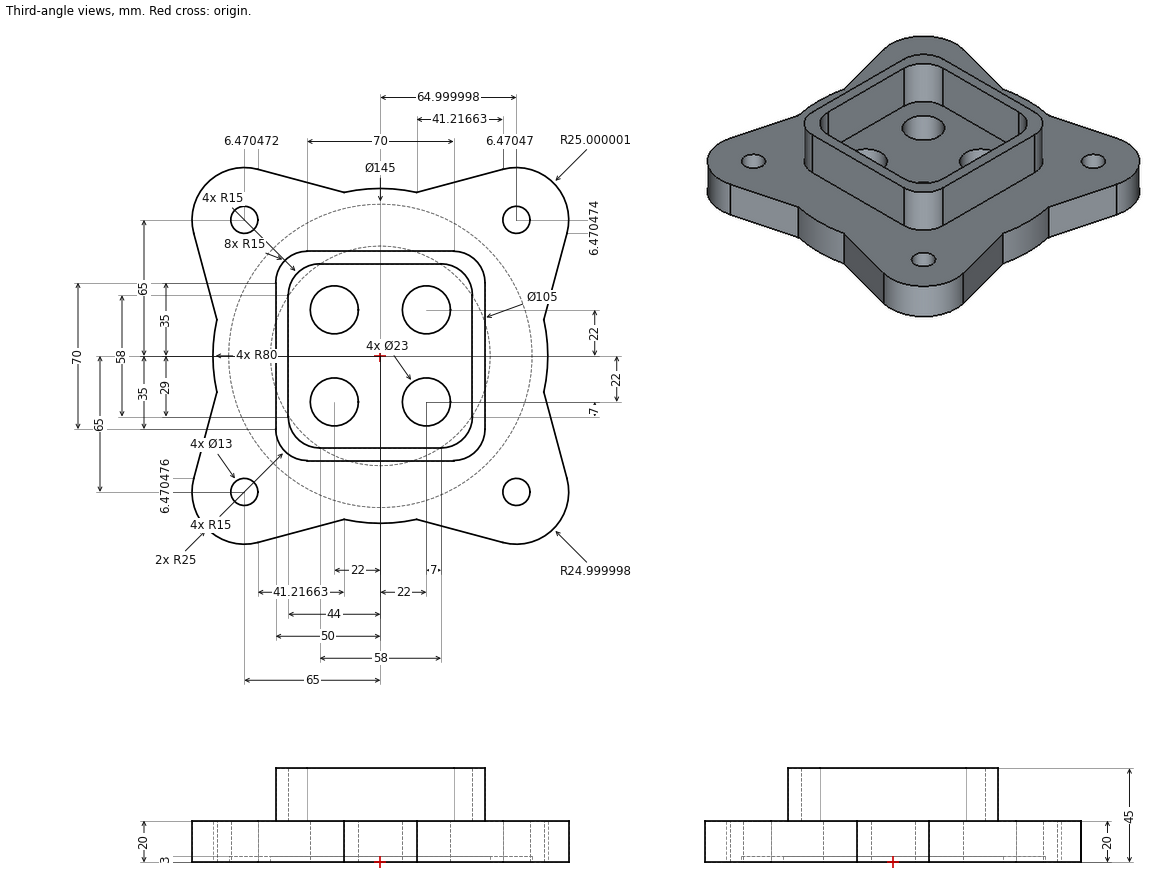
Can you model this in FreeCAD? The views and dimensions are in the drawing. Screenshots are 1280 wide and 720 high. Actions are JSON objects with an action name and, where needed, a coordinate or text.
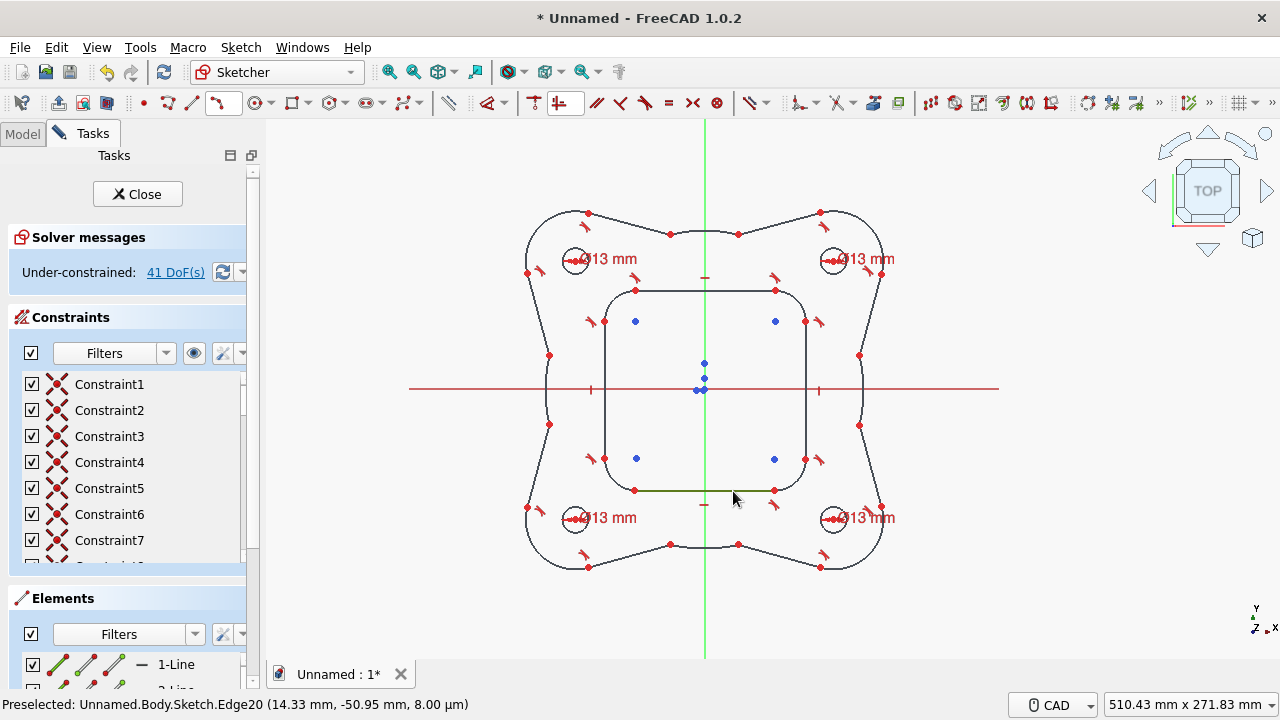
{"action": "left_click", "coordinate": [608, 473]}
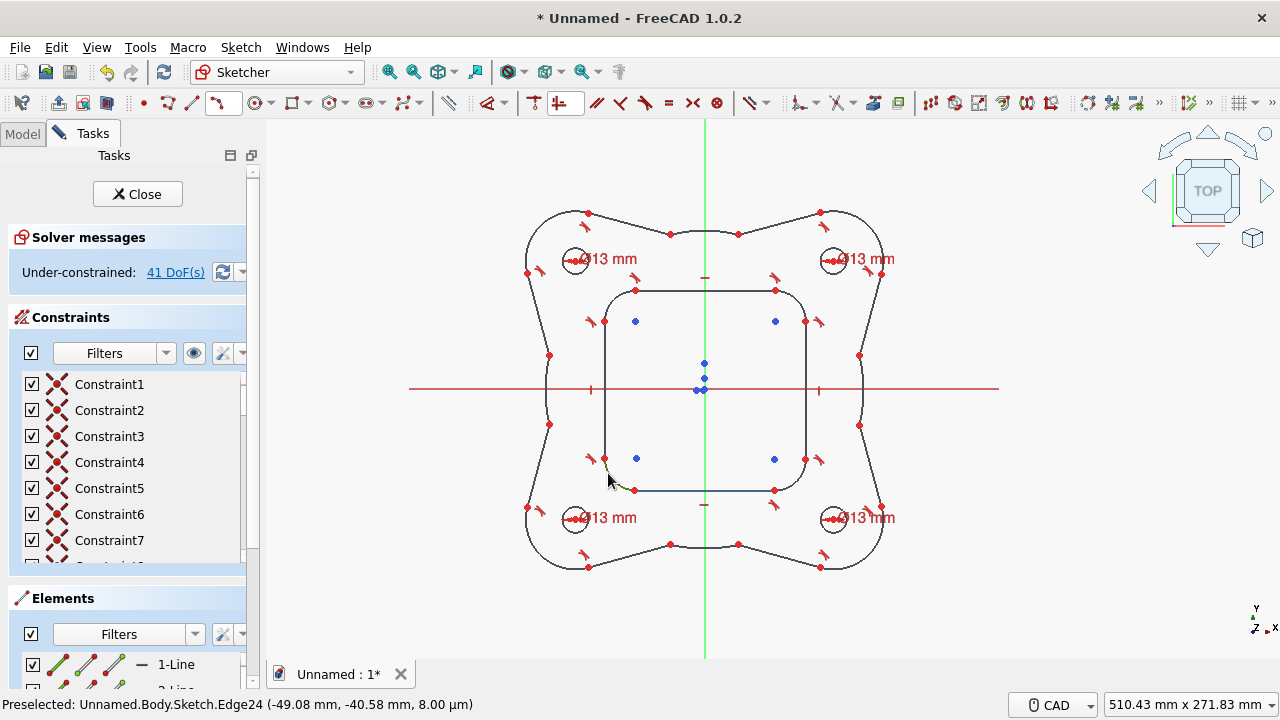
{"action": "left_click", "coordinate": [646, 104]}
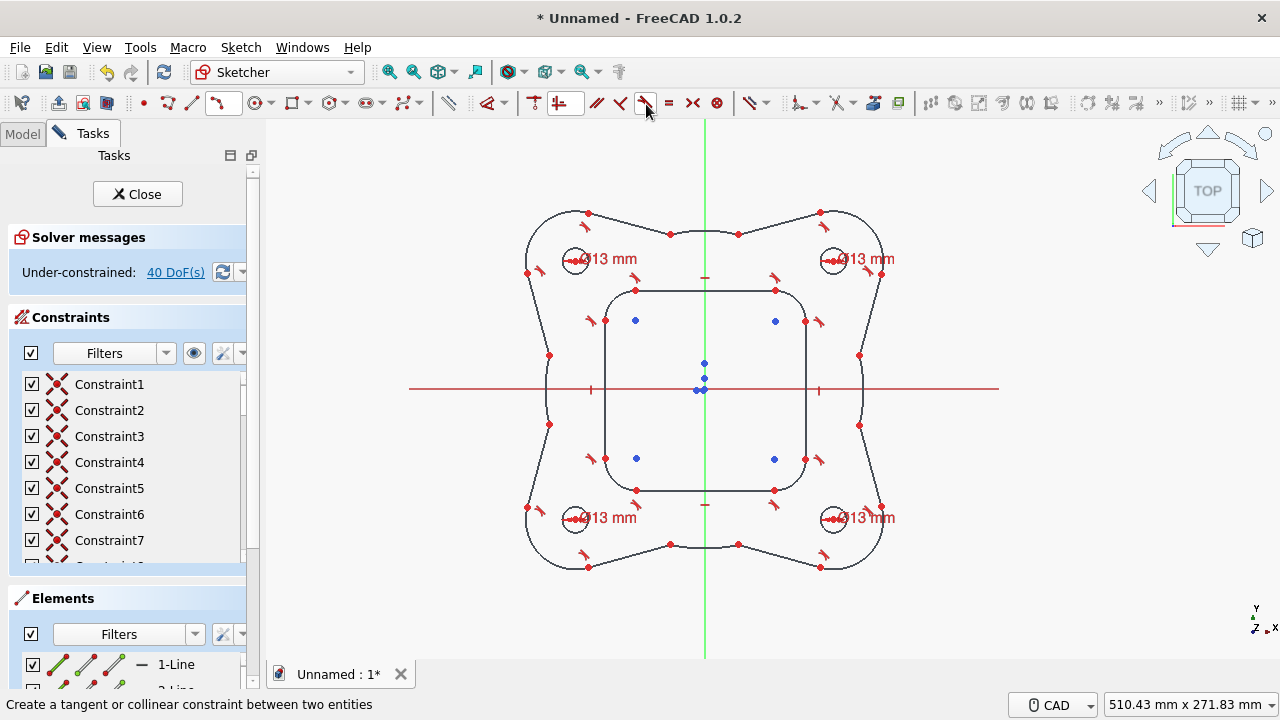
{"action": "left_click", "coordinate": [546, 377]}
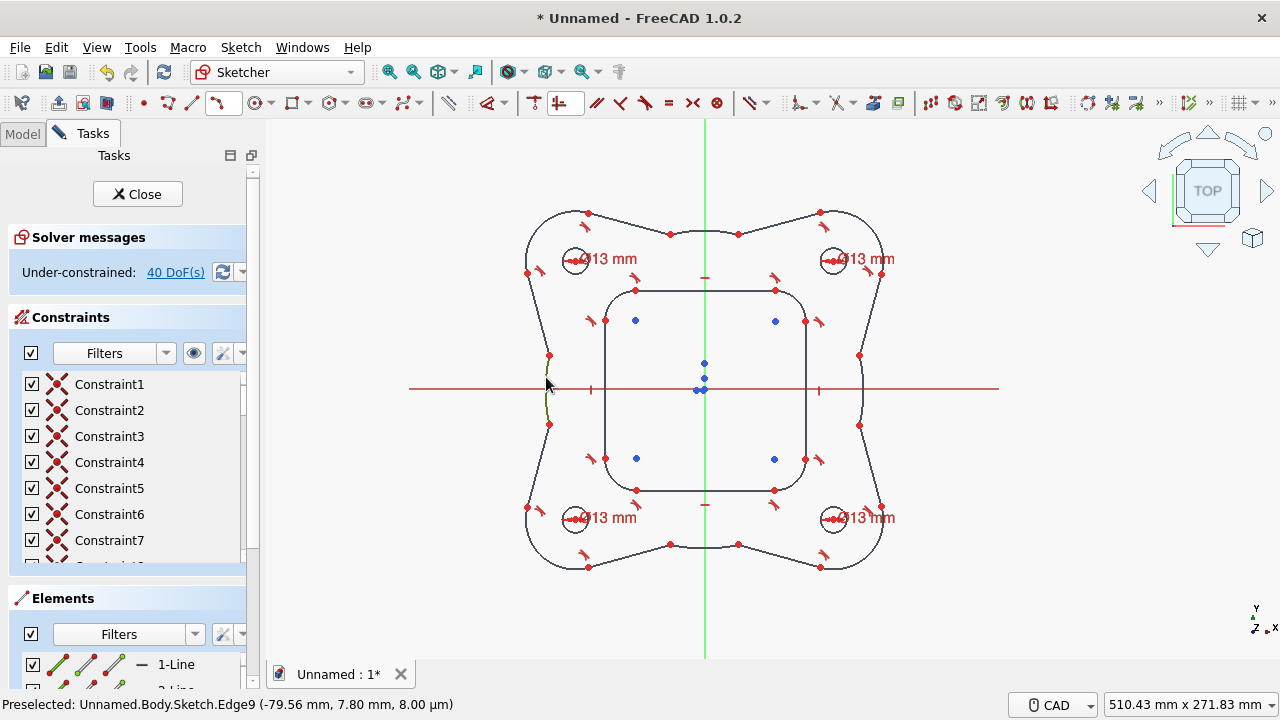
{"action": "left_click", "coordinate": [691, 548]}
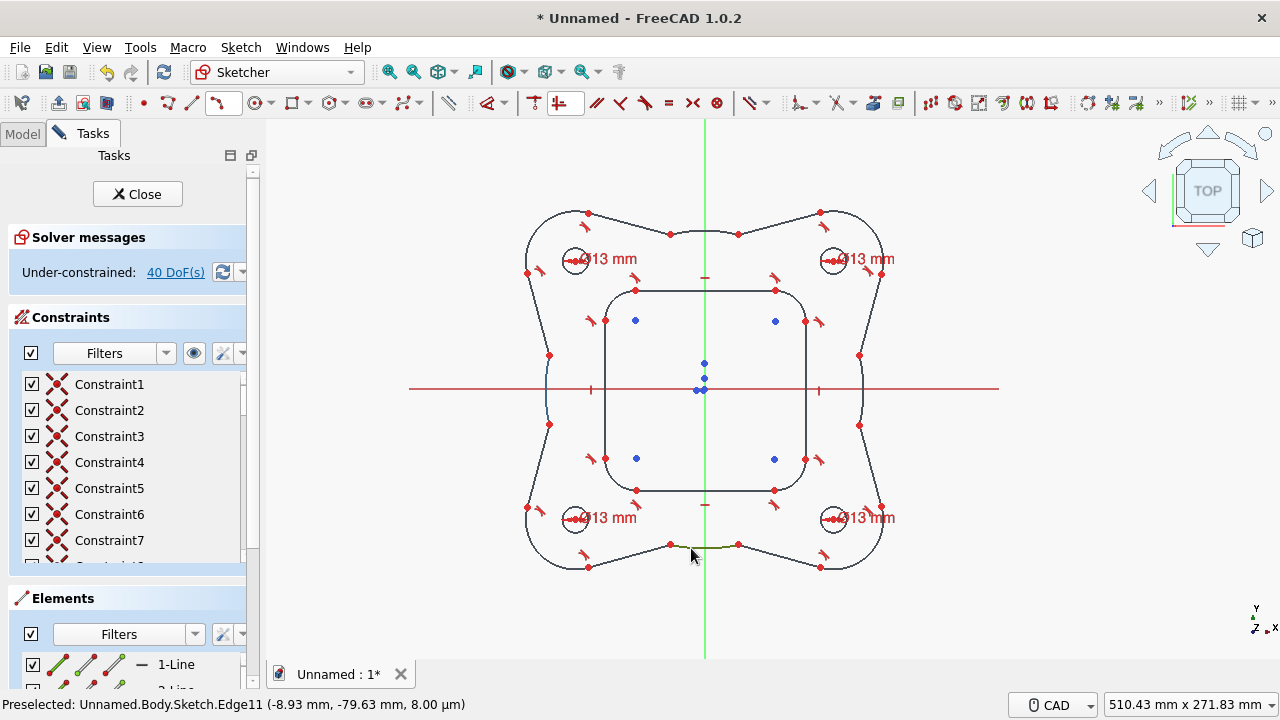
{"action": "key", "text": "c"}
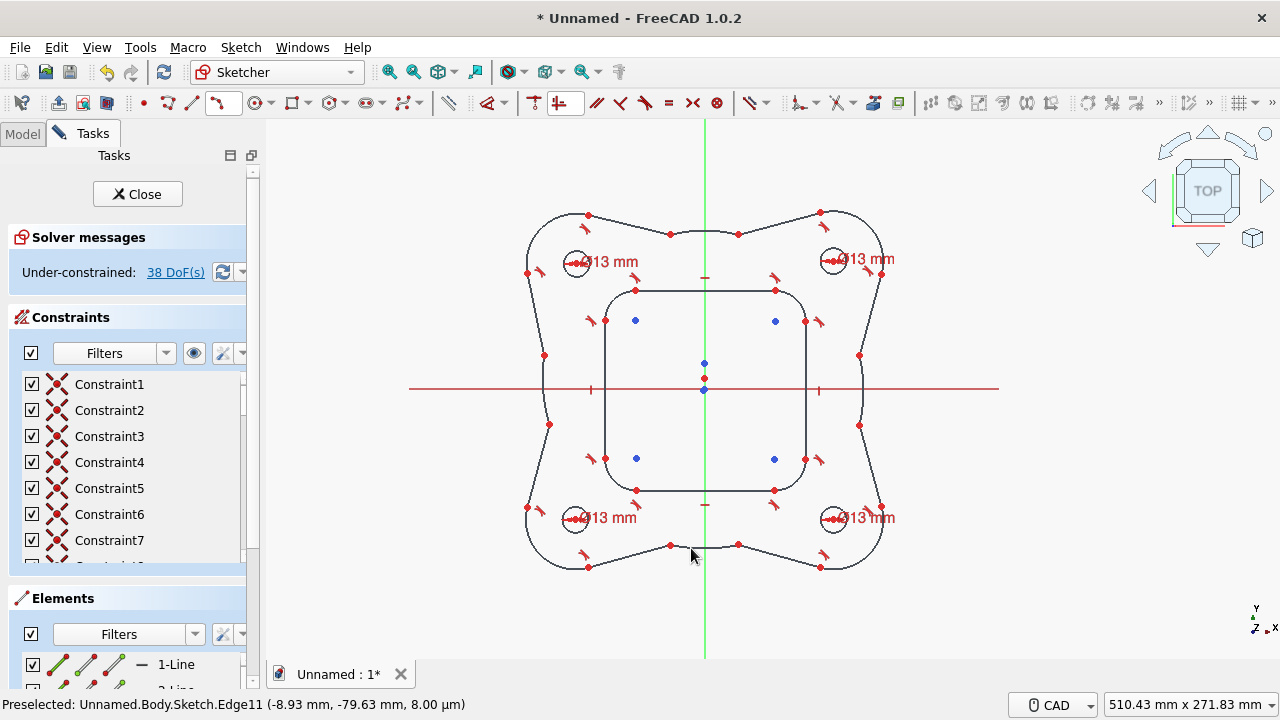
{"action": "left_click", "coordinate": [543, 377]}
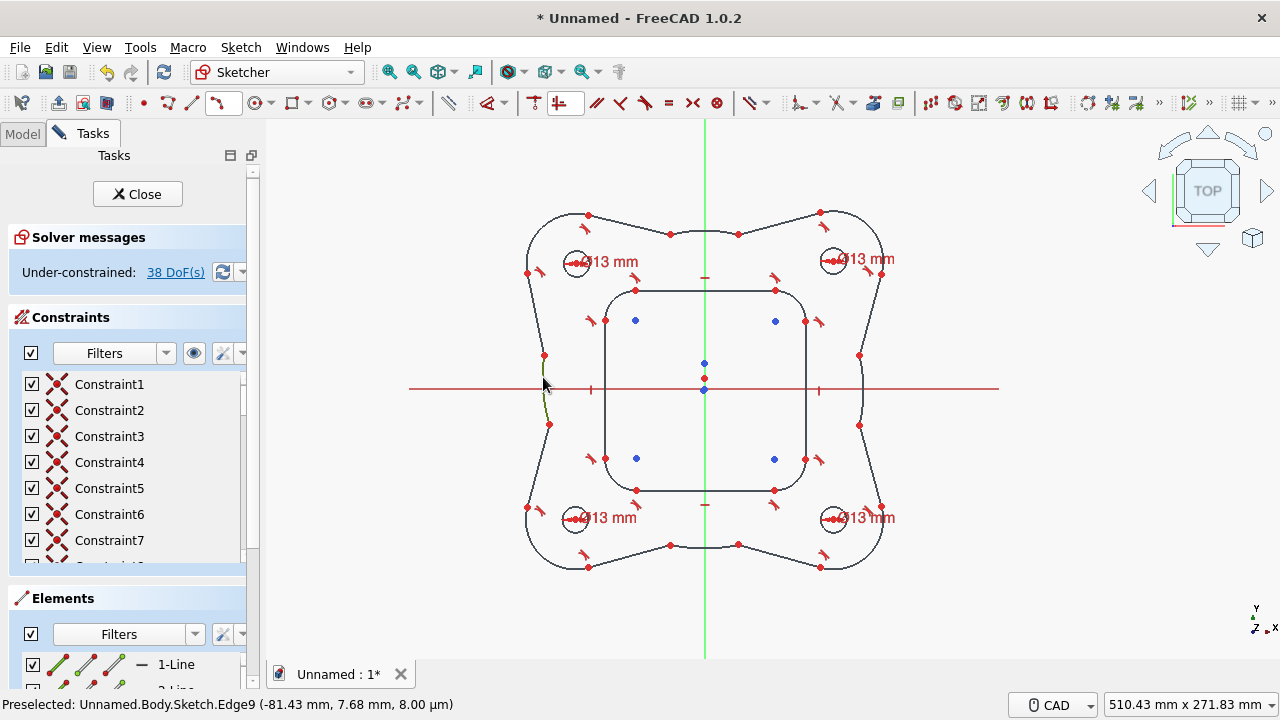
{"action": "left_click", "coordinate": [863, 404]}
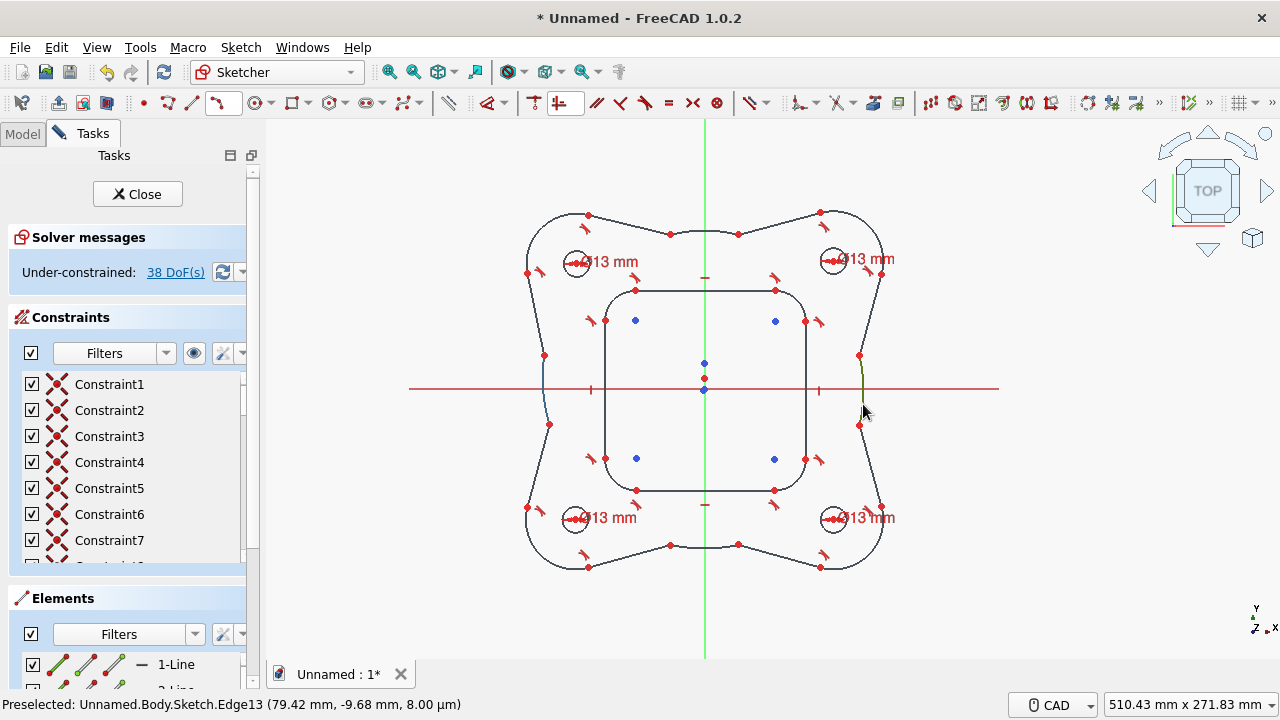
{"action": "left_click", "coordinate": [534, 104]}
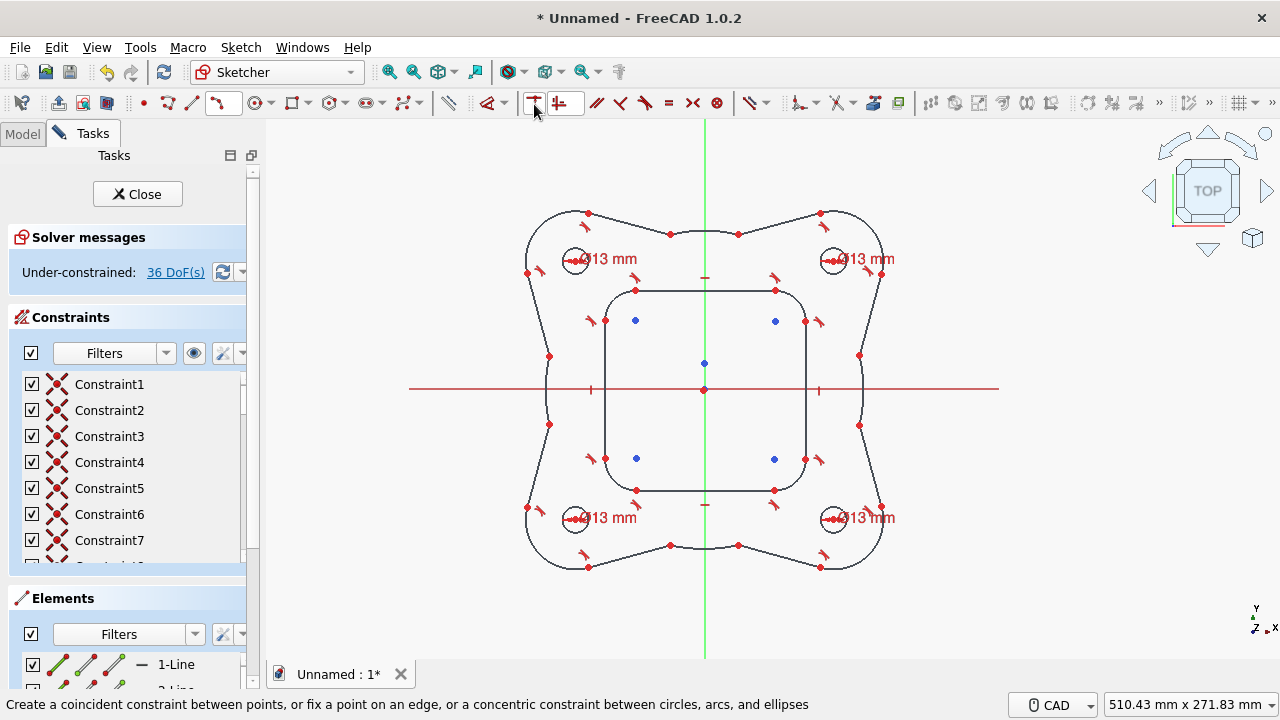
{"action": "left_click", "coordinate": [546, 377]}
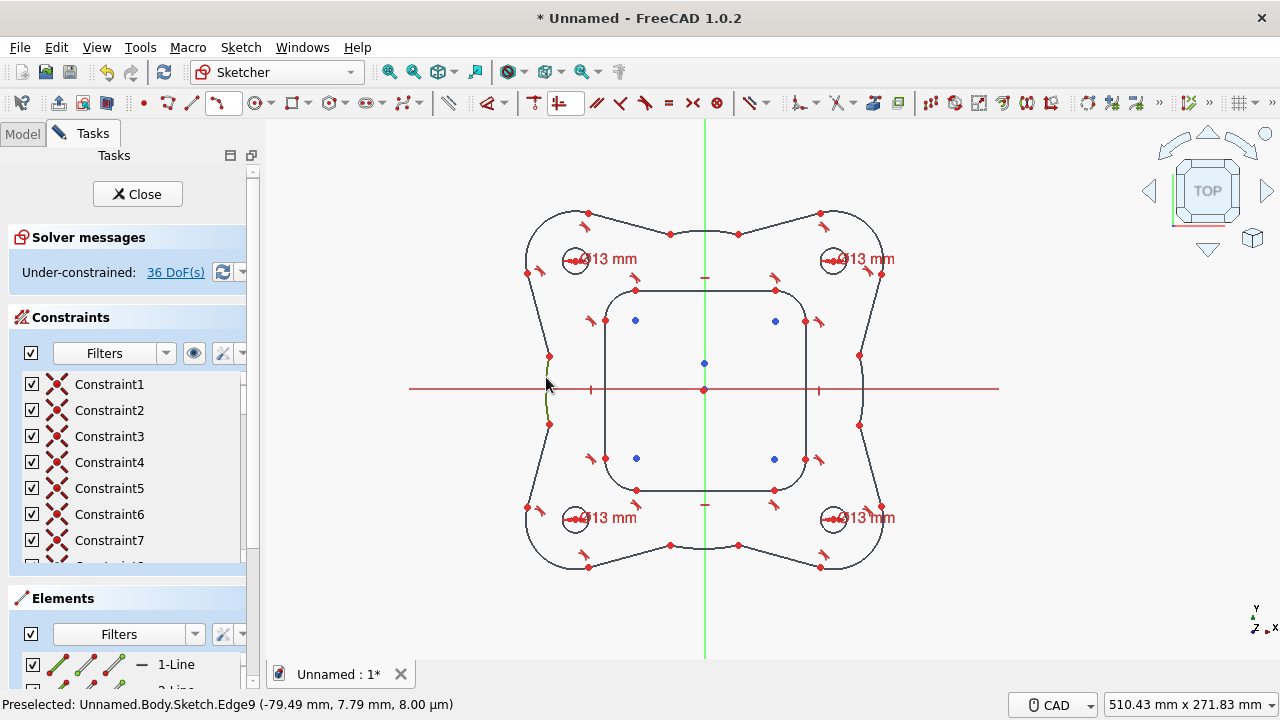
{"action": "left_click", "coordinate": [718, 231]}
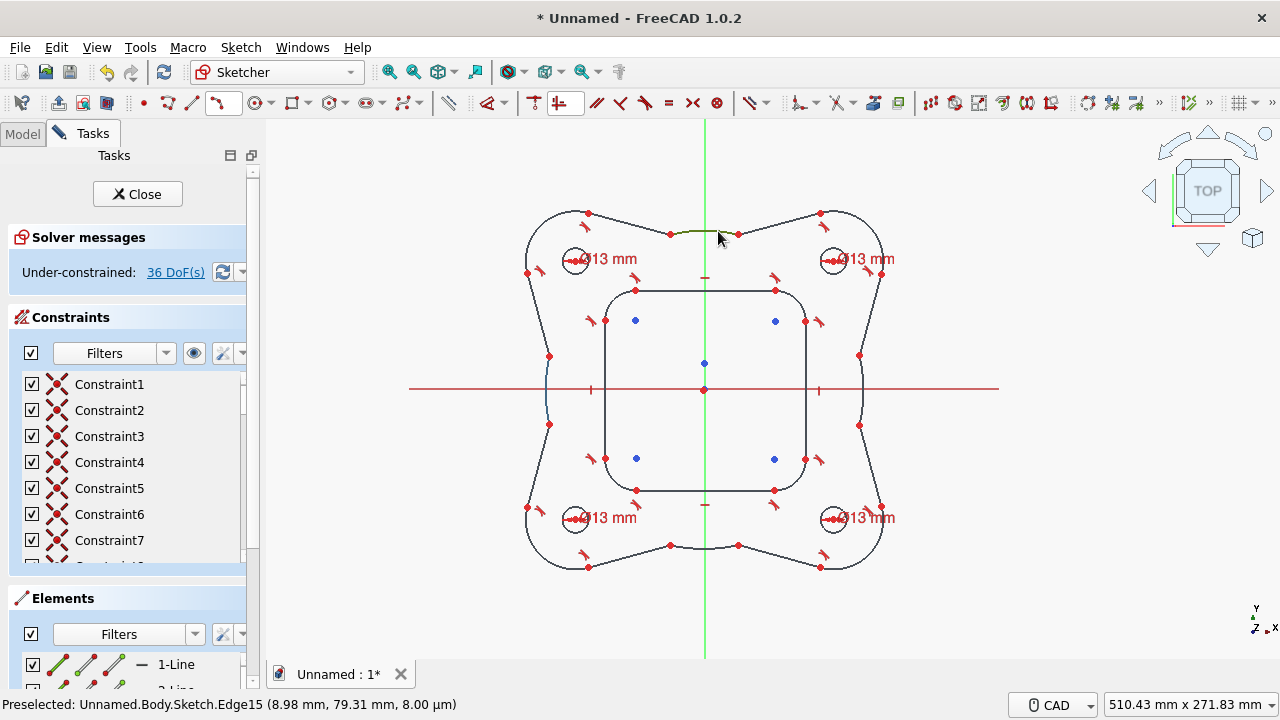
{"action": "key", "text": "c"}